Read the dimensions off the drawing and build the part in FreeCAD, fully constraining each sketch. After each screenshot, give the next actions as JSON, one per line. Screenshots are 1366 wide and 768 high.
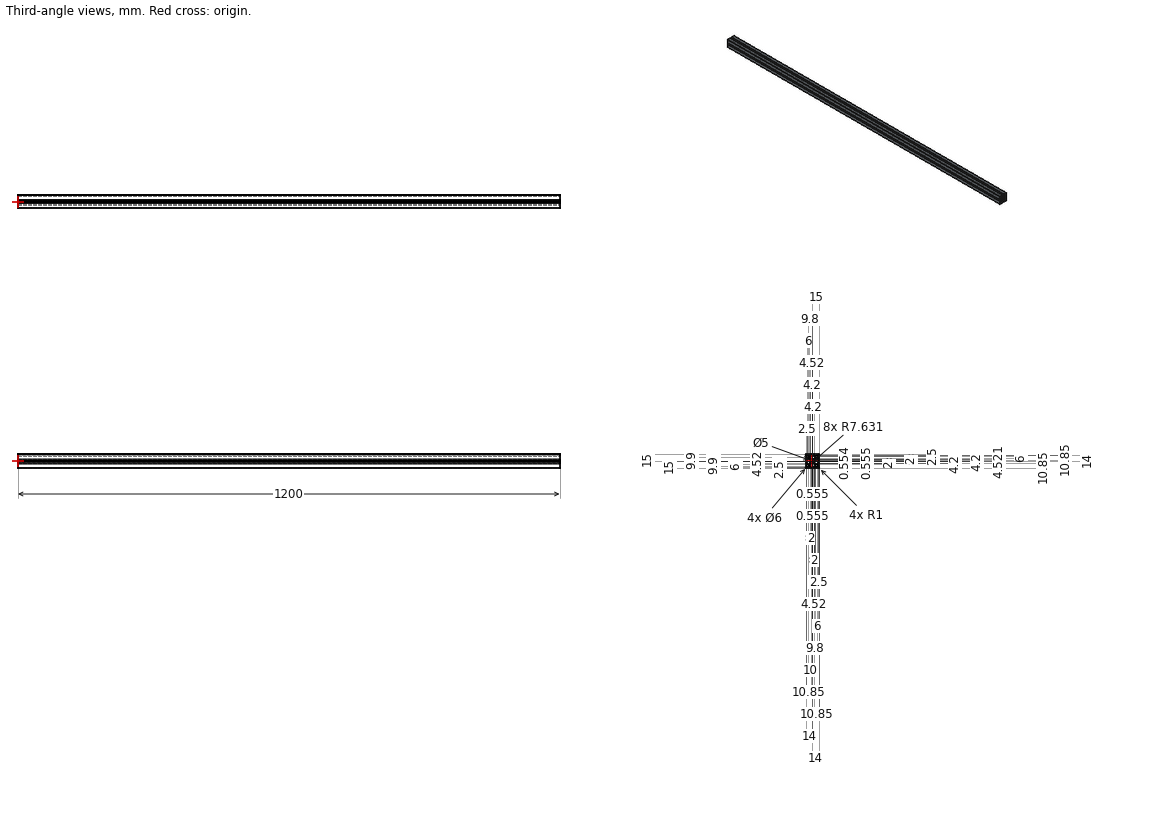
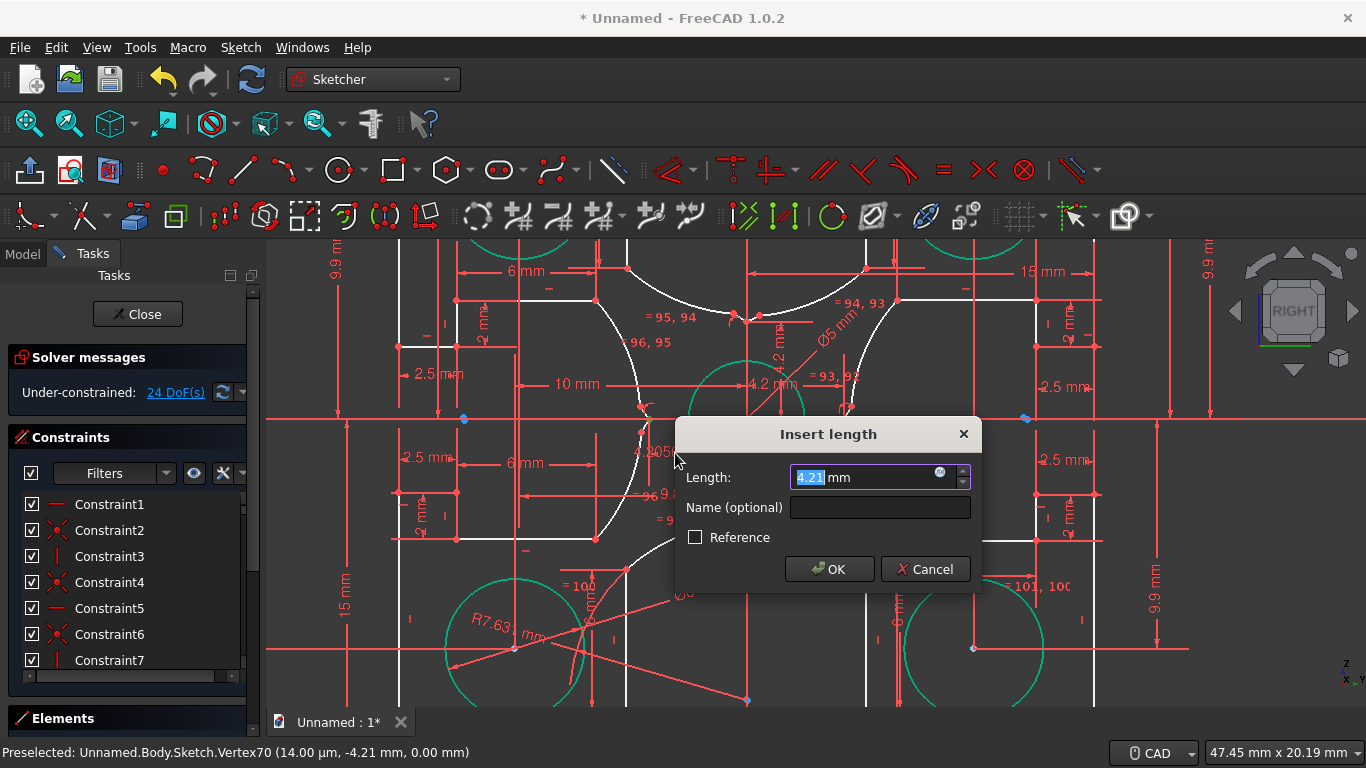
{"action": "type", "text": "4.2"}
{"action": "key", "text": "Return"}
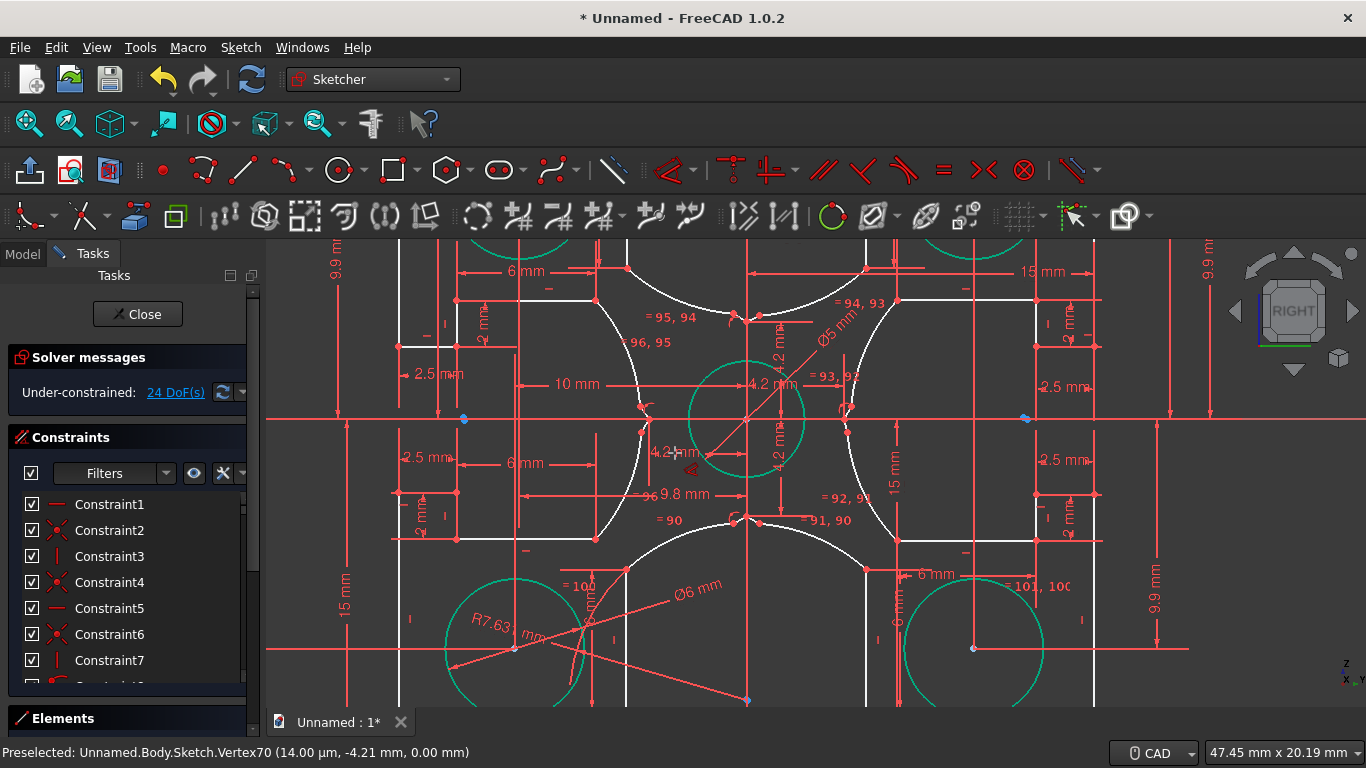
{"action": "scroll", "coordinate": [748, 517], "scroll_direction": "down", "scroll_amount": 4}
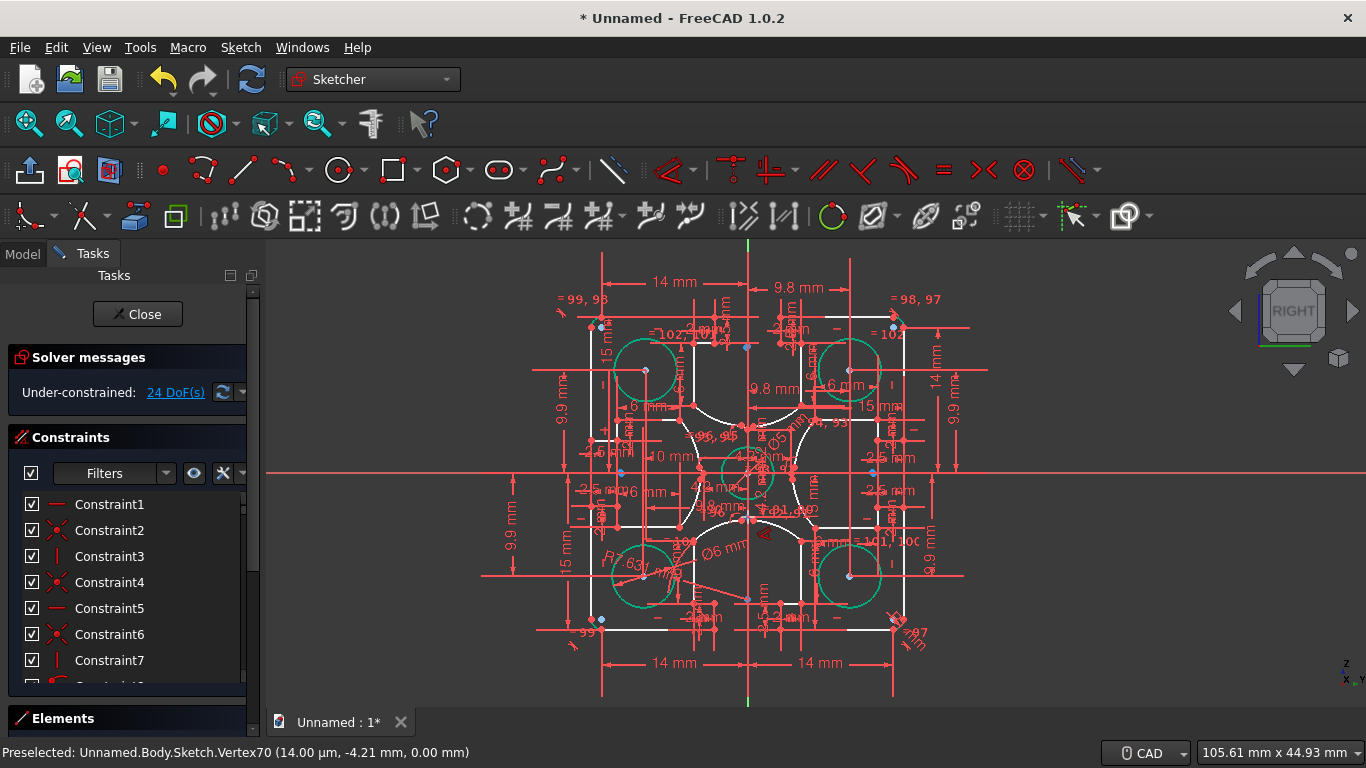
{"action": "left_click", "coordinate": [636, 630]}
{"action": "left_click", "coordinate": [632, 664]}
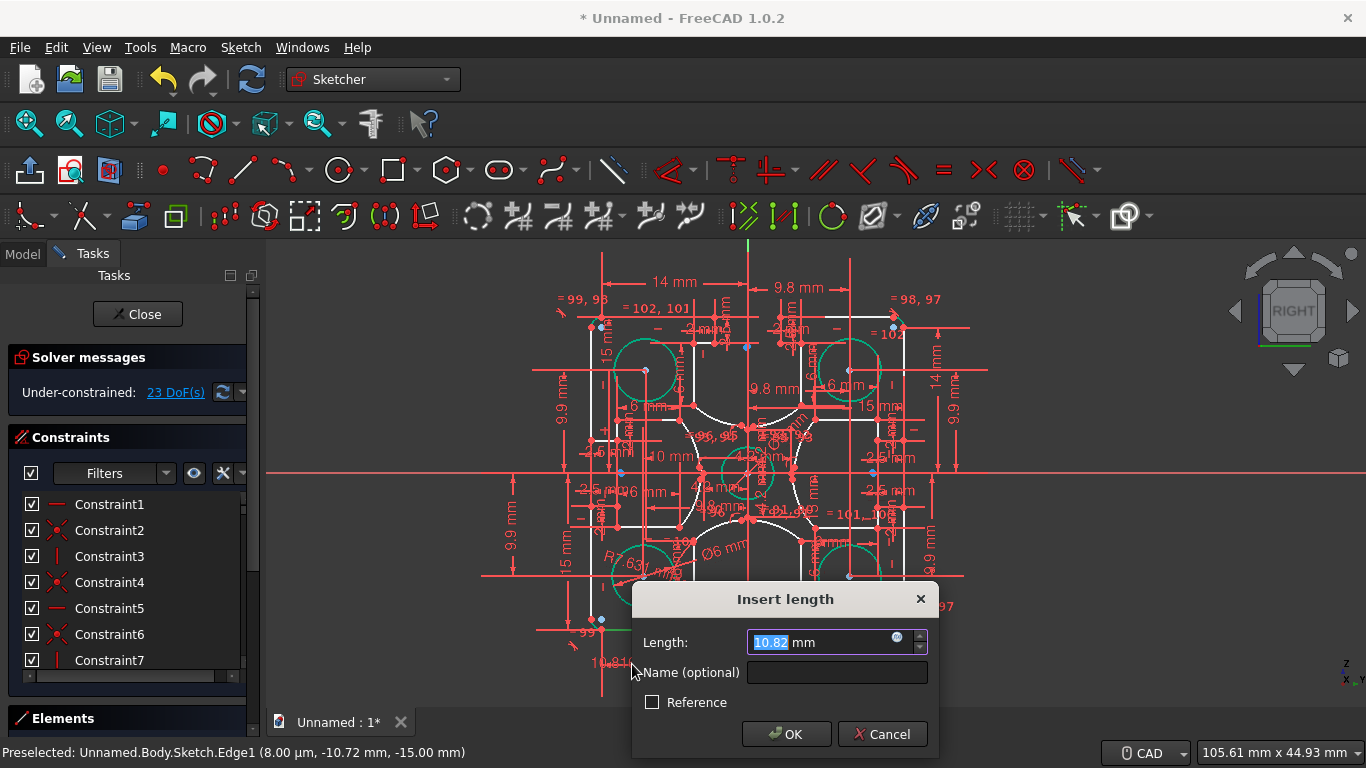
{"action": "type", "text": "10.85"}
{"action": "key", "text": "Return"}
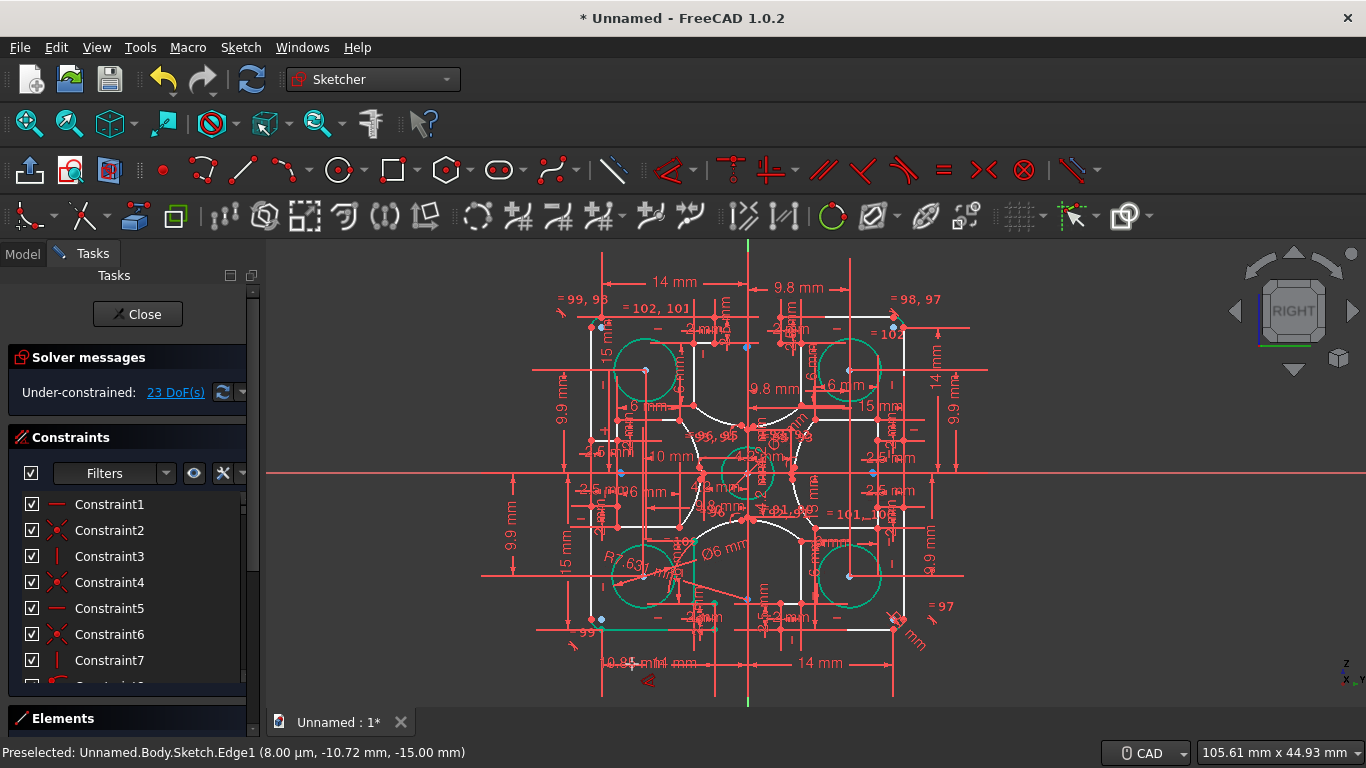
{"action": "left_click", "coordinate": [814, 630]}
{"action": "left_click", "coordinate": [863, 664]}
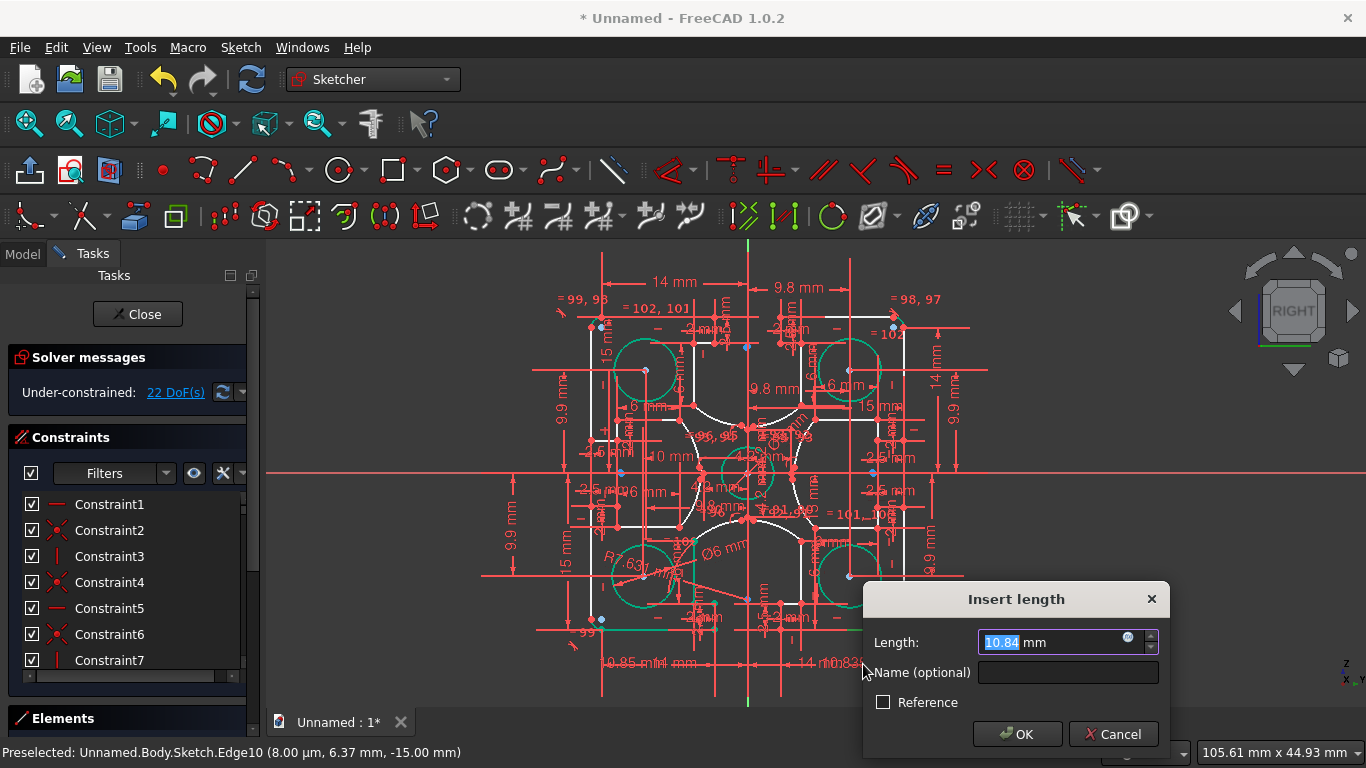
{"action": "type", "text": "10.85"}
{"action": "key", "text": "Return"}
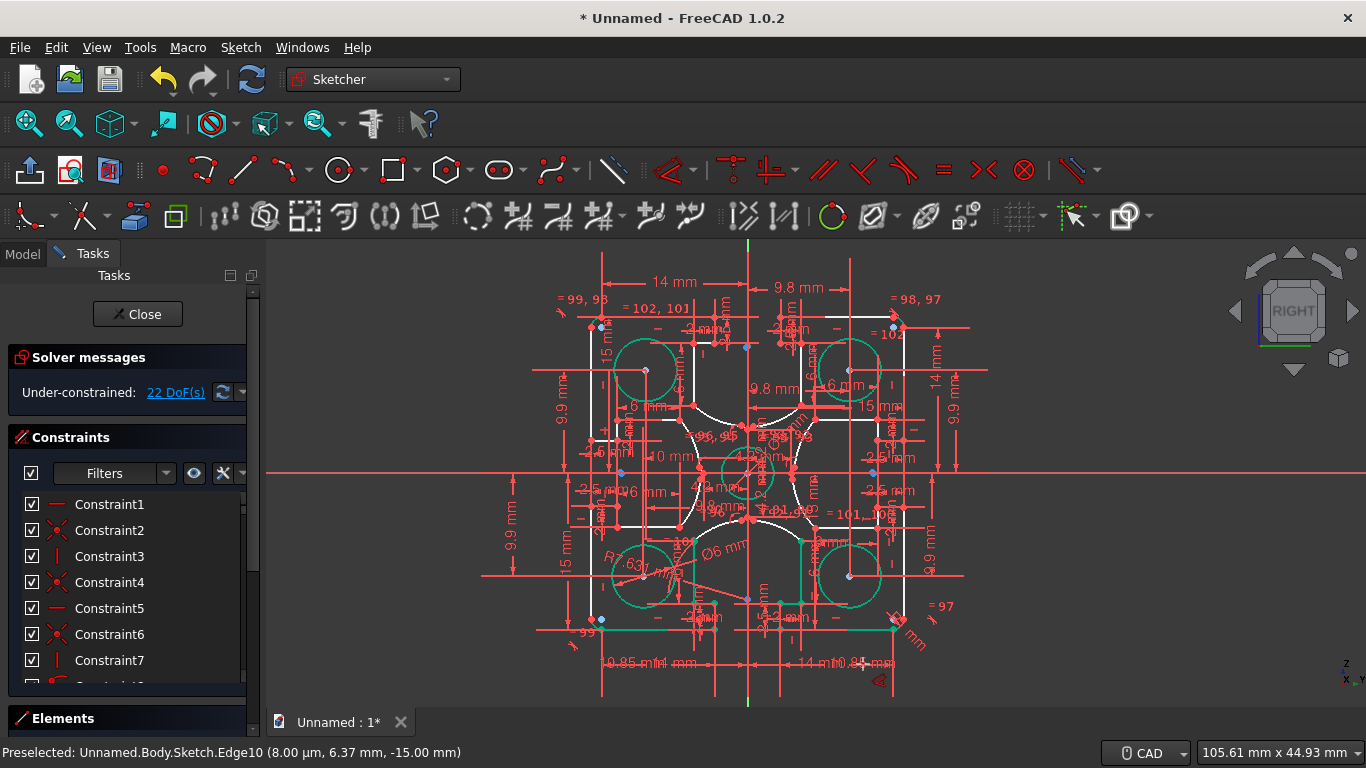
{"action": "left_click", "coordinate": [904, 586]}
{"action": "left_click", "coordinate": [938, 589]}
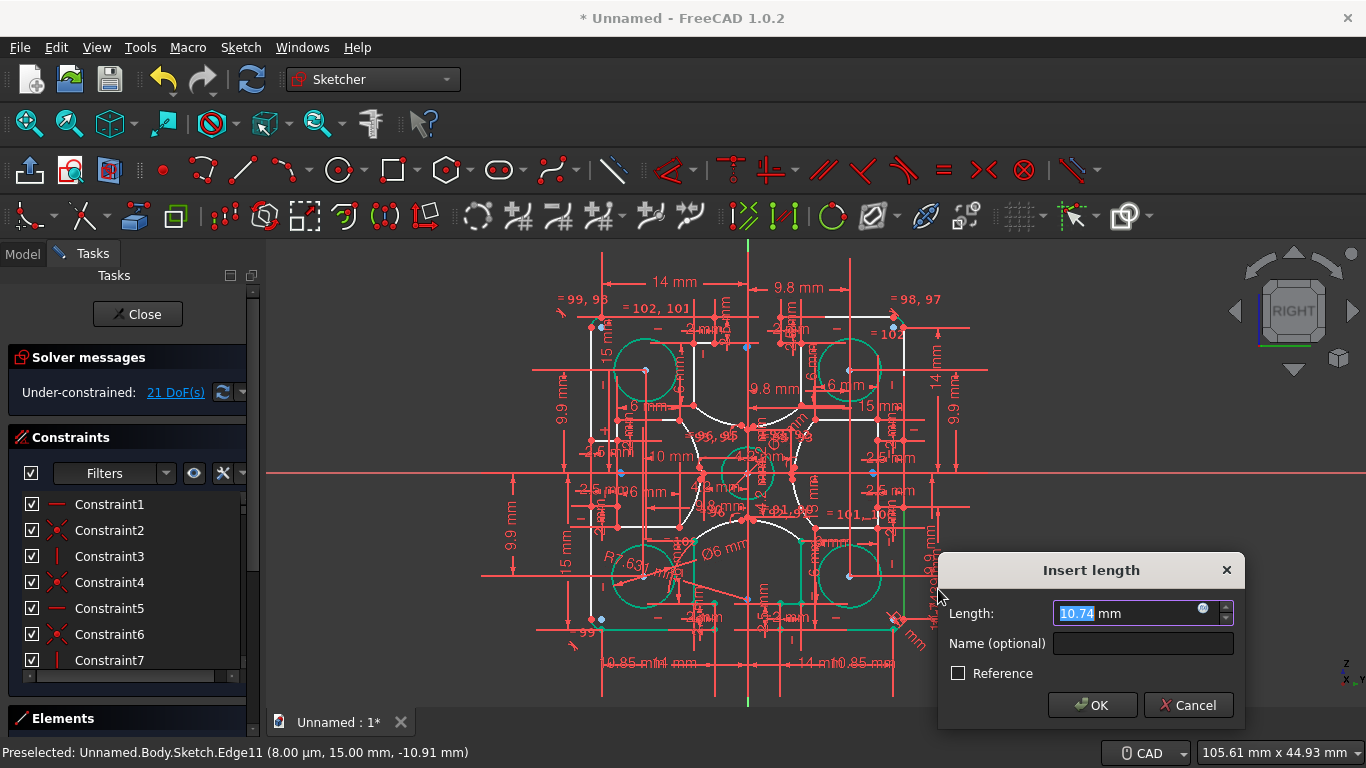
{"action": "type", "text": "10.85"}
{"action": "key", "text": "Return"}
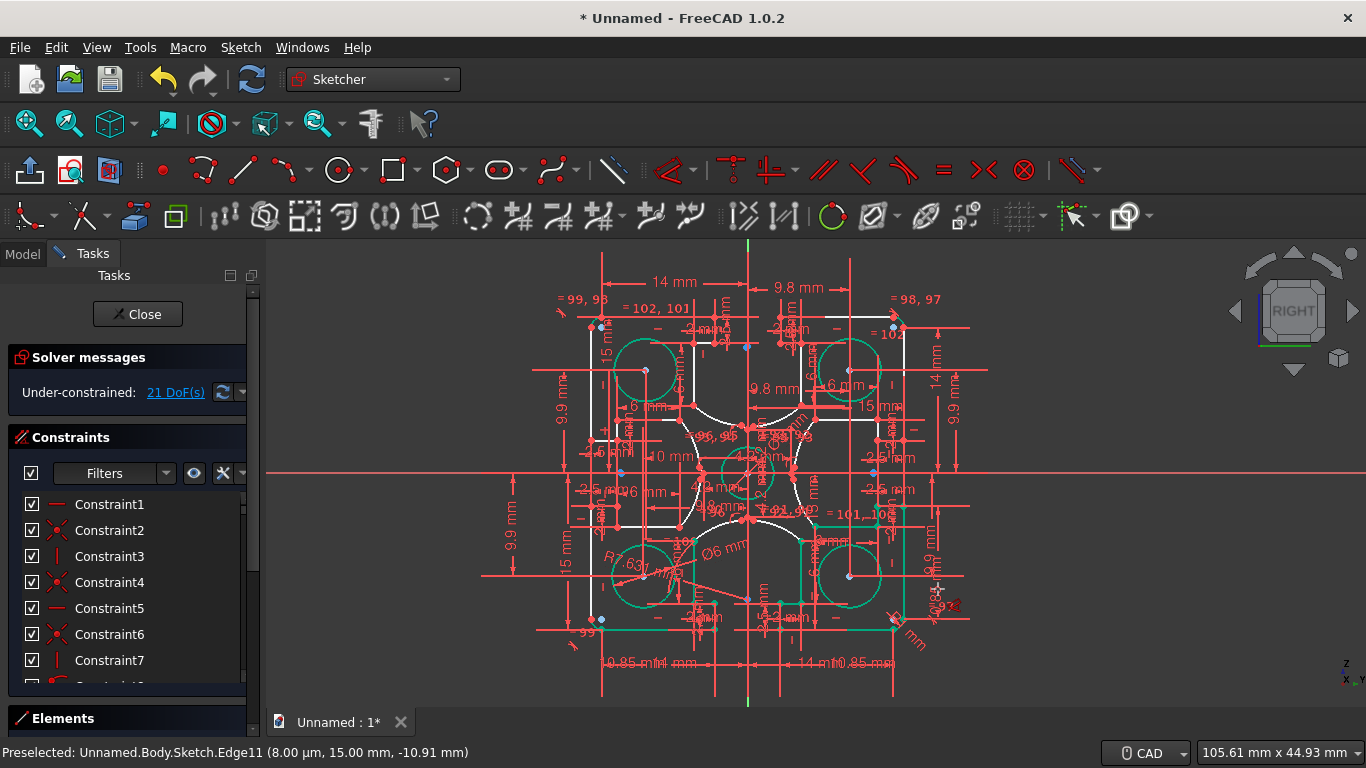
{"action": "left_click", "coordinate": [904, 407]}
{"action": "left_click", "coordinate": [986, 424]}